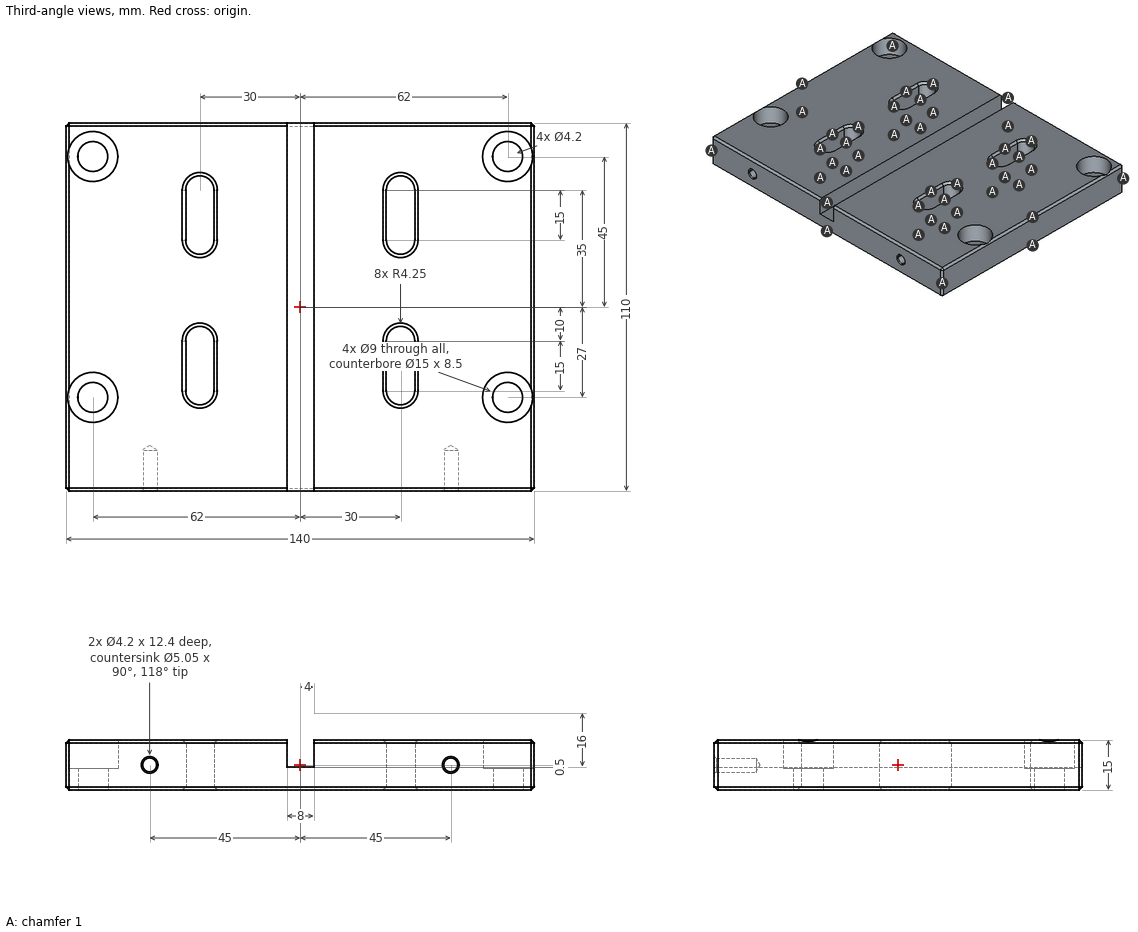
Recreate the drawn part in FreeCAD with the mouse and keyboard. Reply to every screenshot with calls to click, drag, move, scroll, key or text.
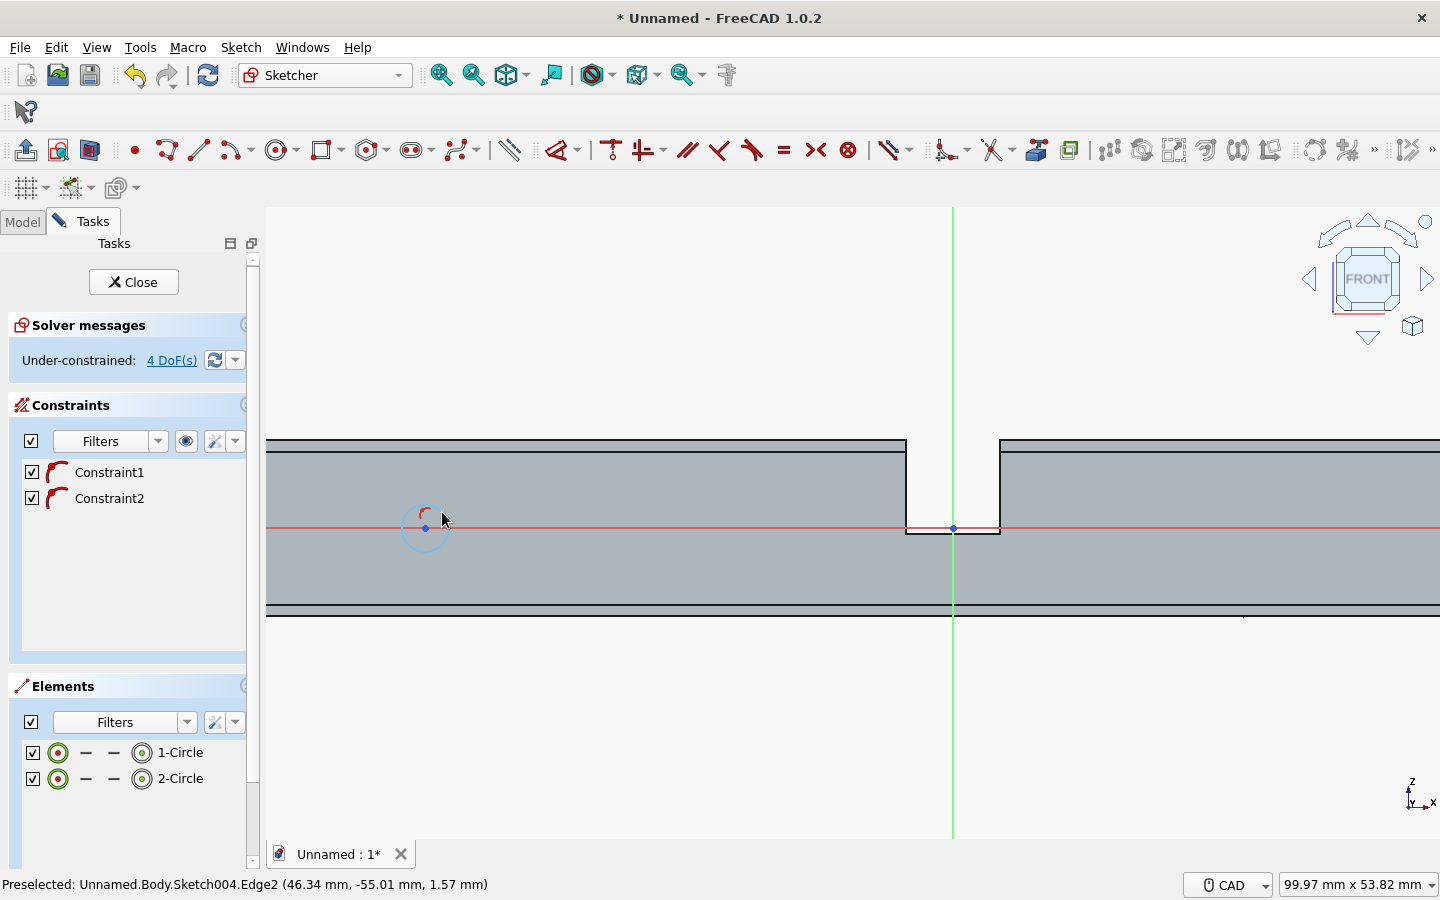
click(442, 512)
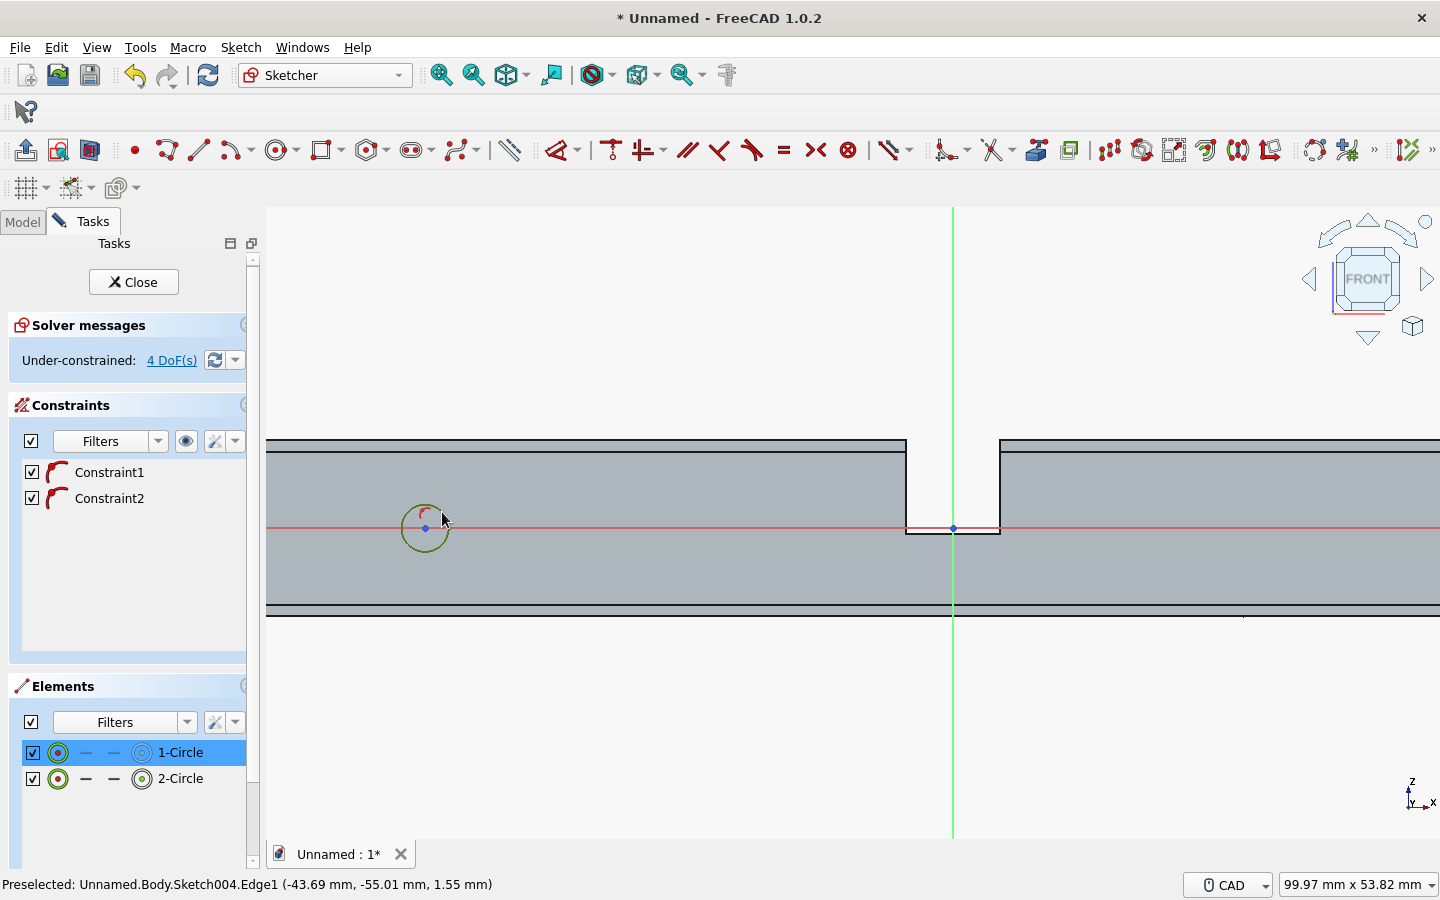
scroll(442, 512, down, 2)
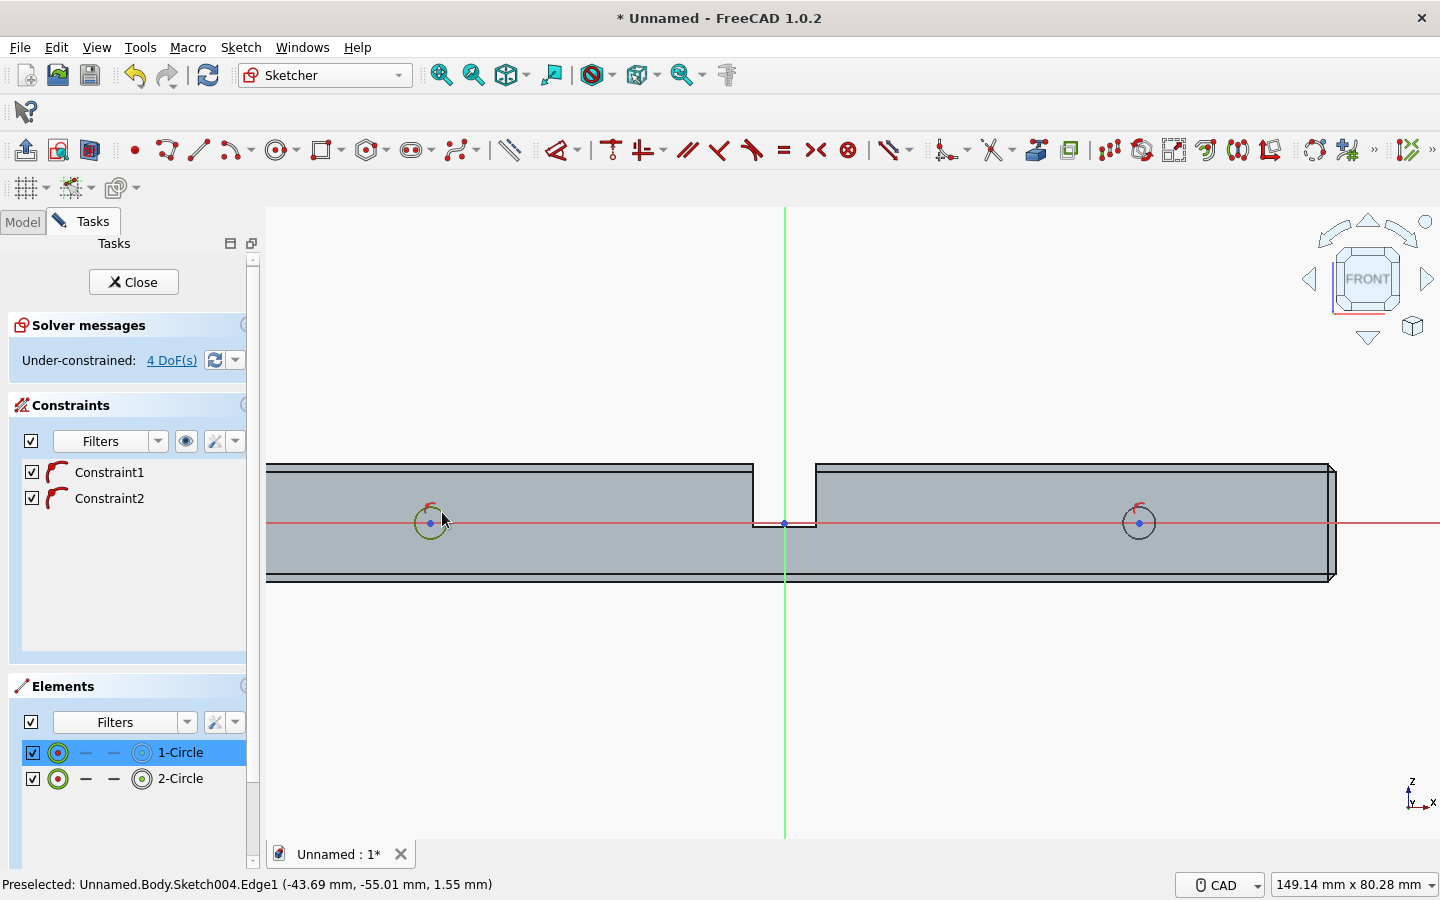
click(1151, 512)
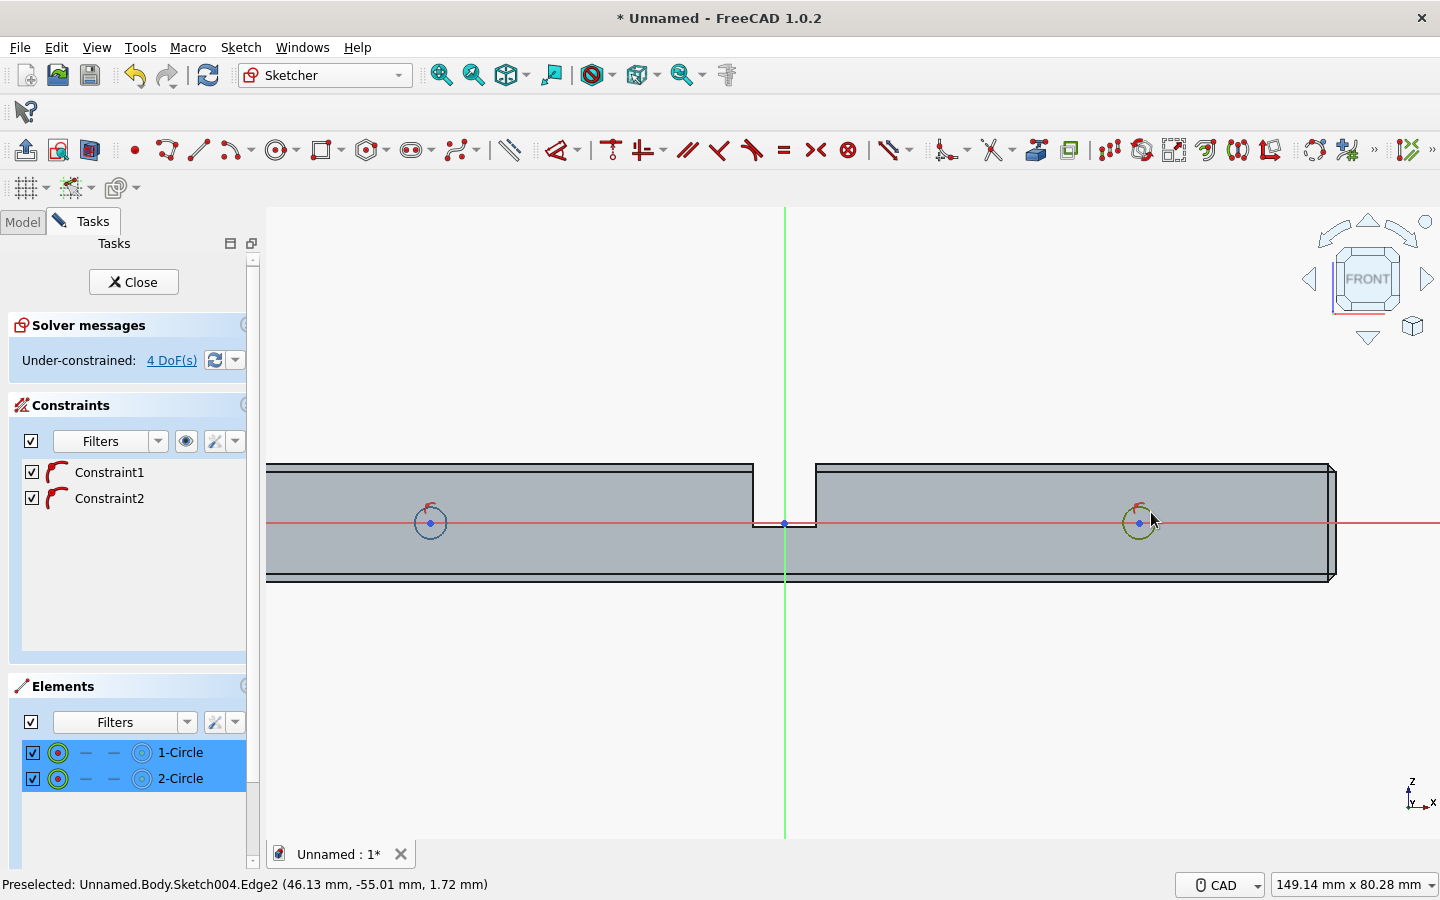
key(e)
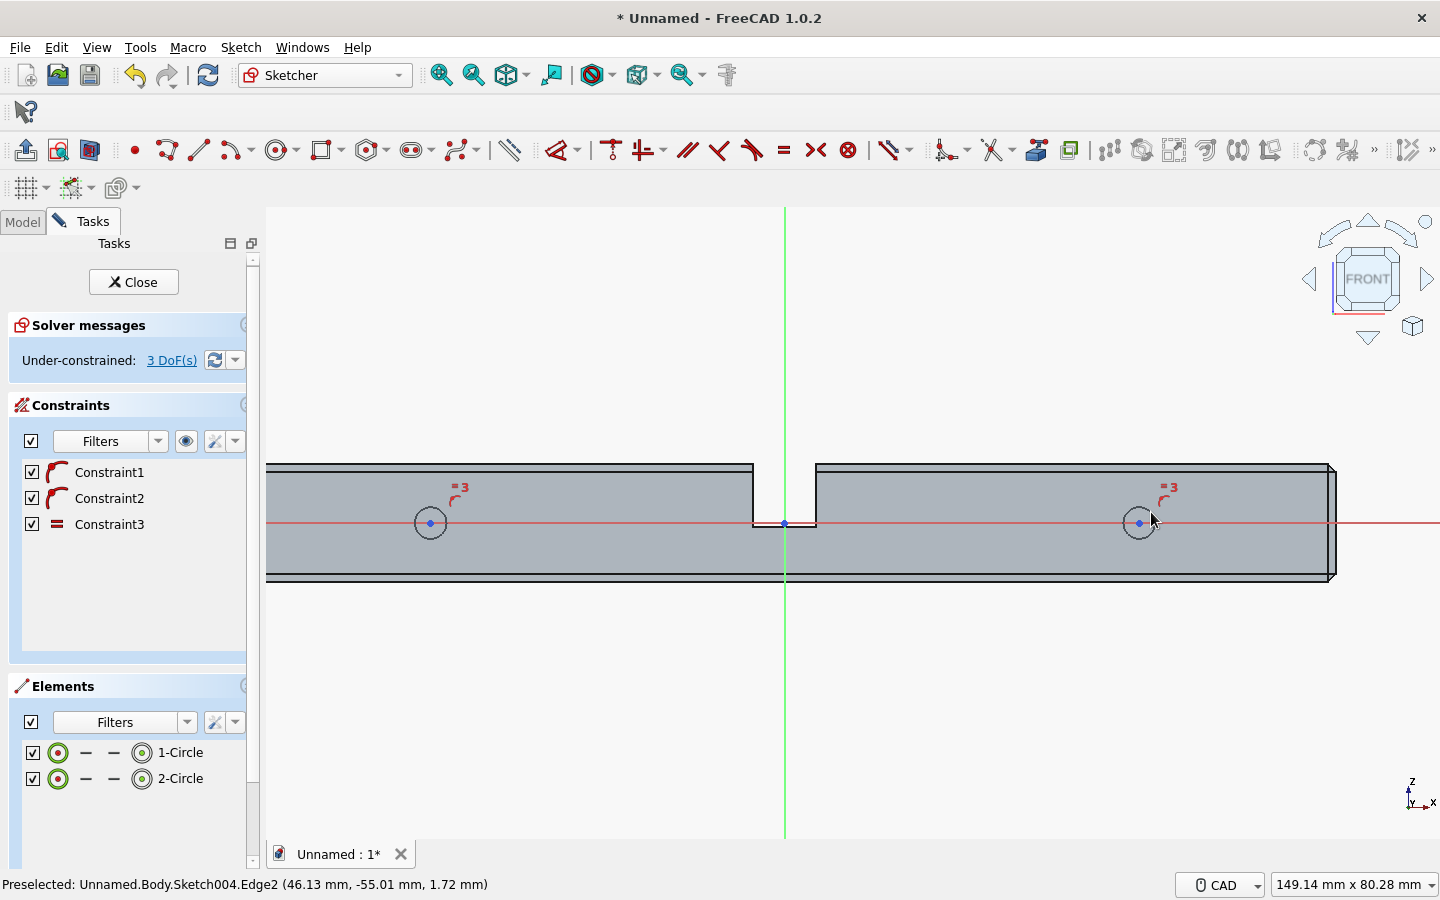
click(556, 150)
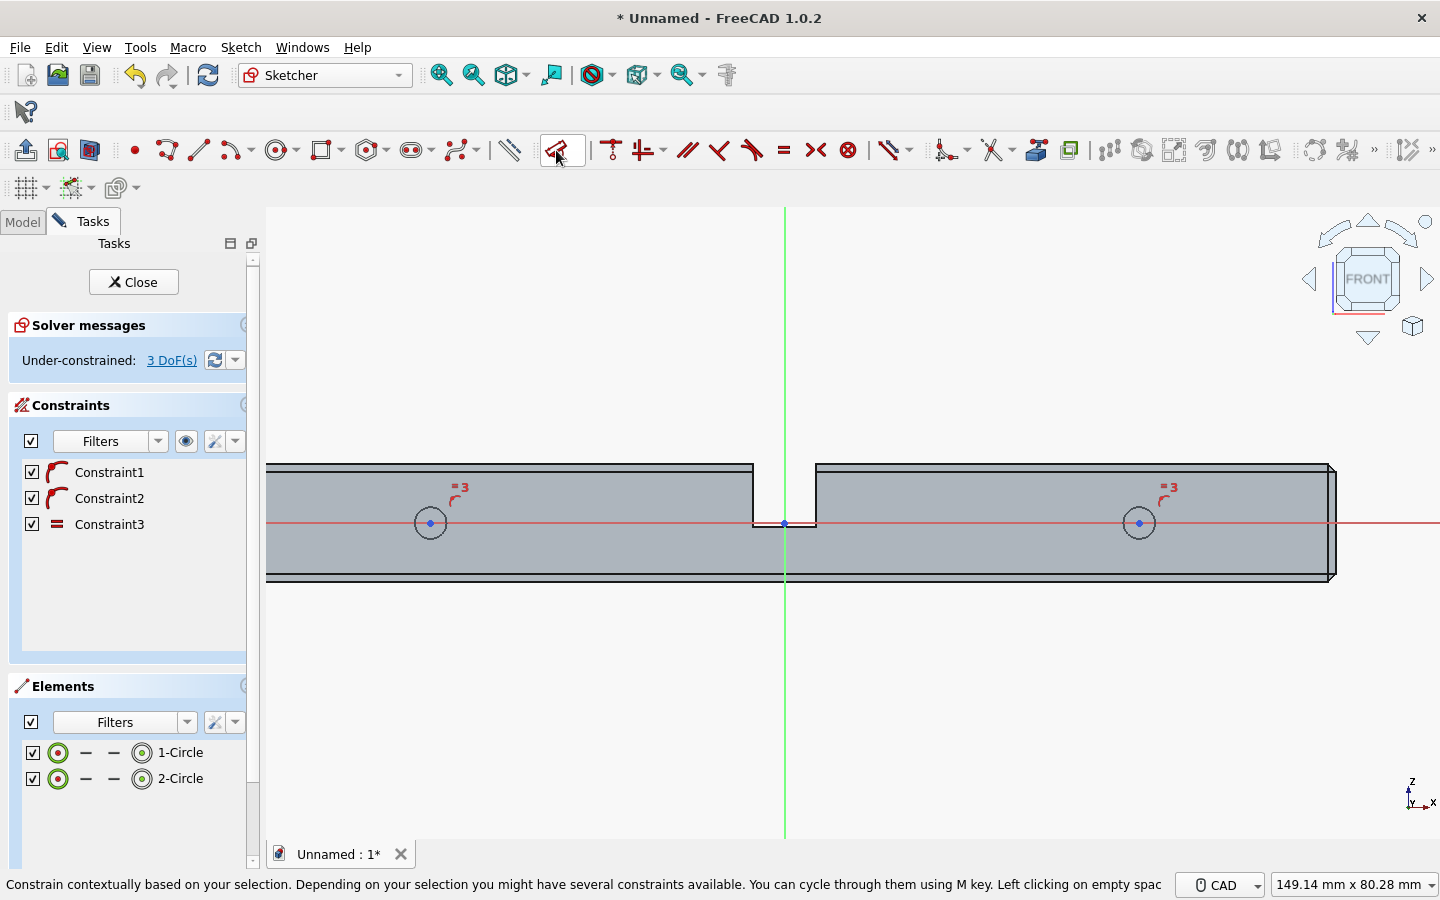
scroll(442, 512, up, 2)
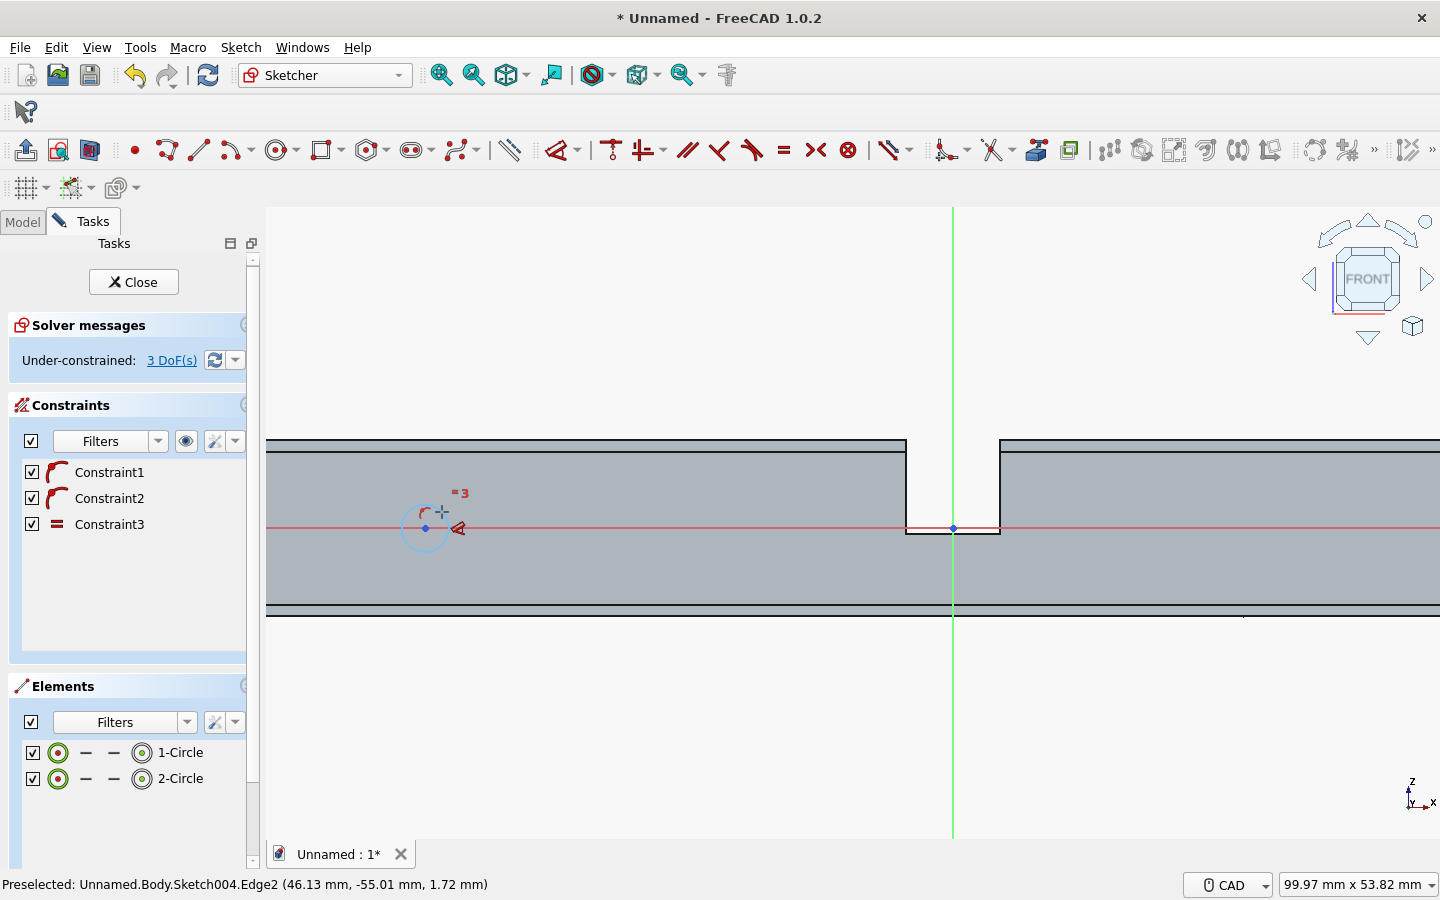
click(442, 512)
click(465, 490)